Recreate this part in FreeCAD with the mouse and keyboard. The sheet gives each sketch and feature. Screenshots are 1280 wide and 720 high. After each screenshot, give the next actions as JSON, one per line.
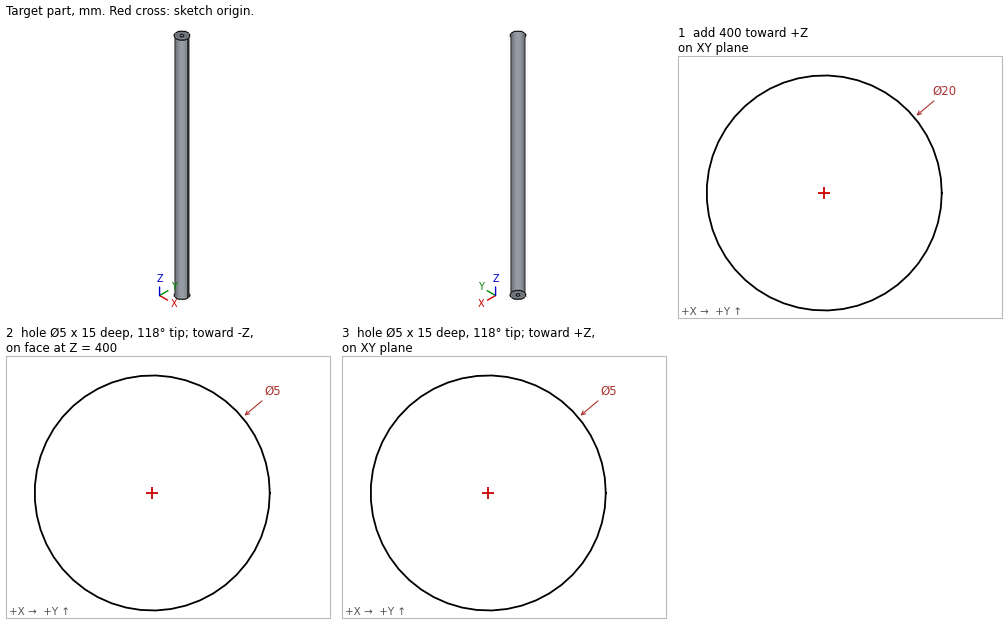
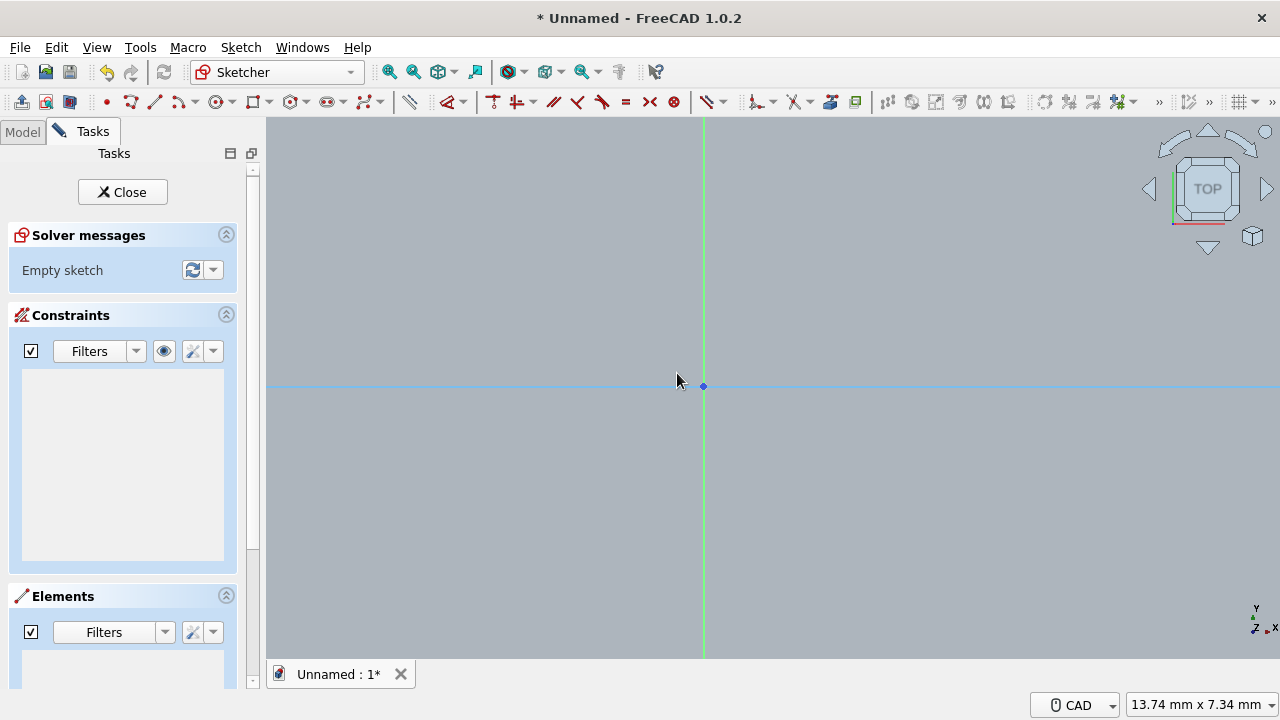
{"action": "key", "text": "g c"}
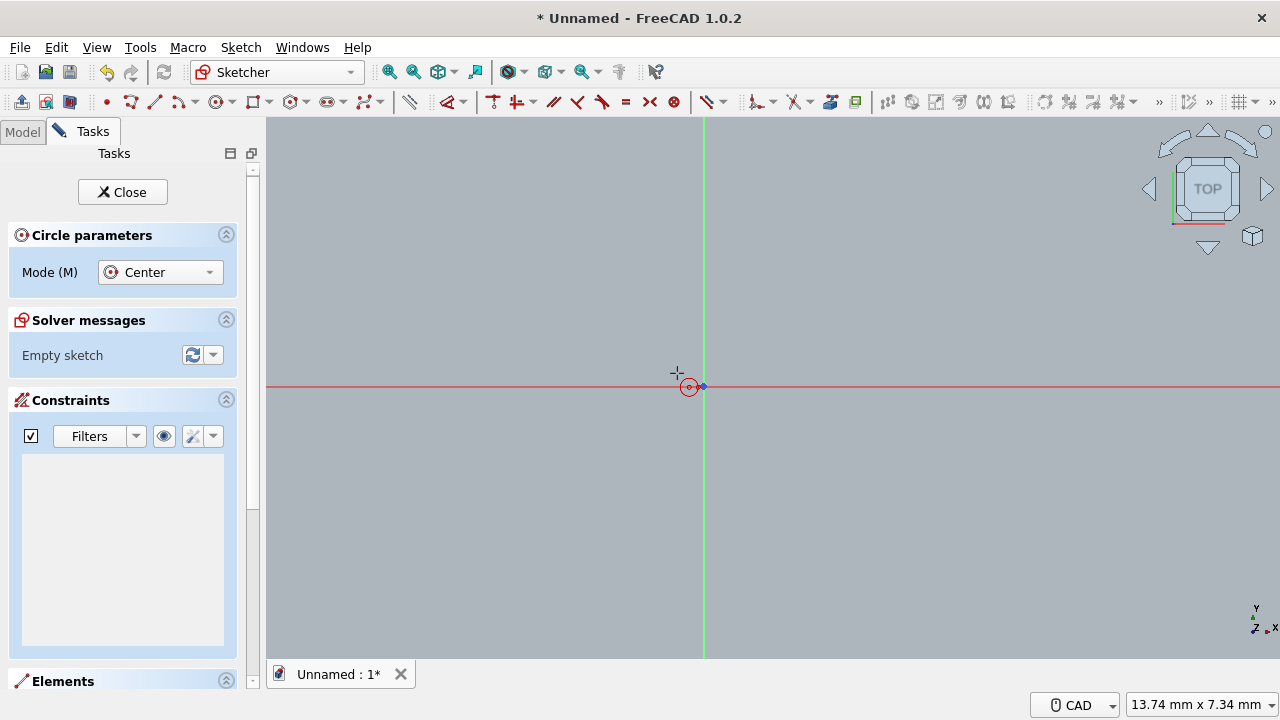
{"action": "left_click", "coordinate": [704, 387]}
{"action": "mouse_move", "coordinate": [834, 257]}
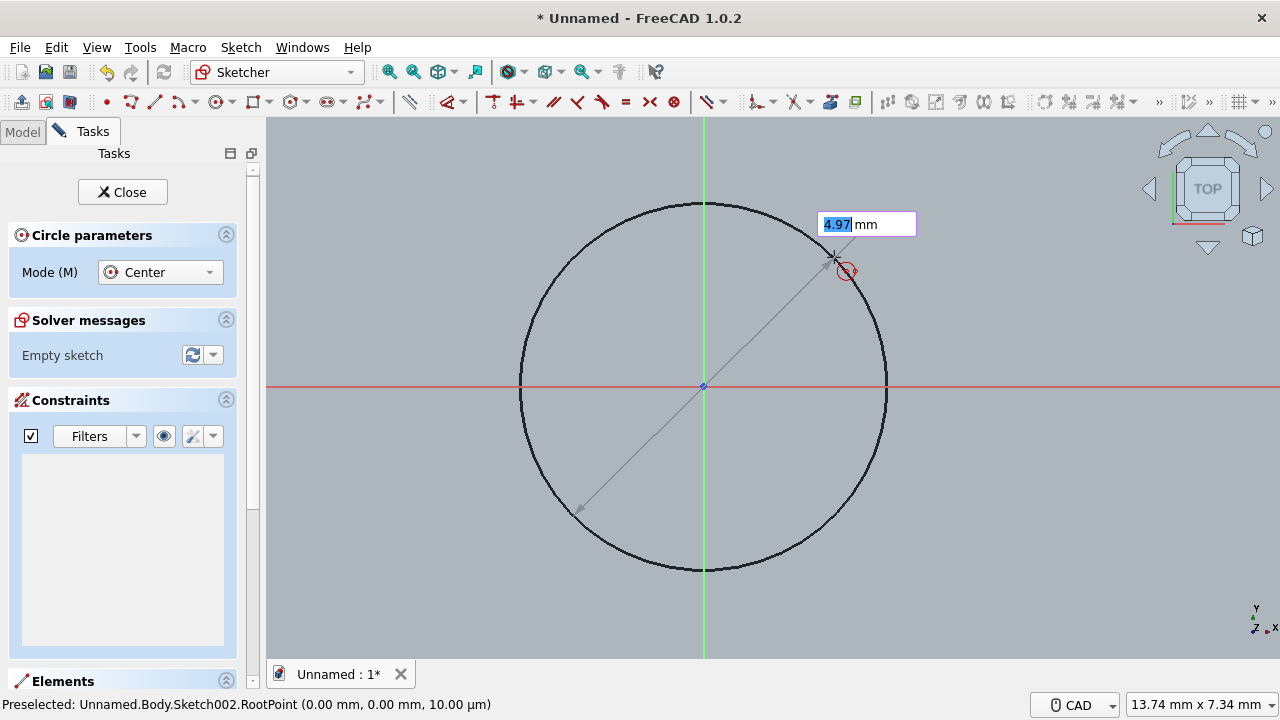
{"action": "type", "text": "5"}
{"action": "key", "text": "Return"}
{"action": "key", "text": "Escape"}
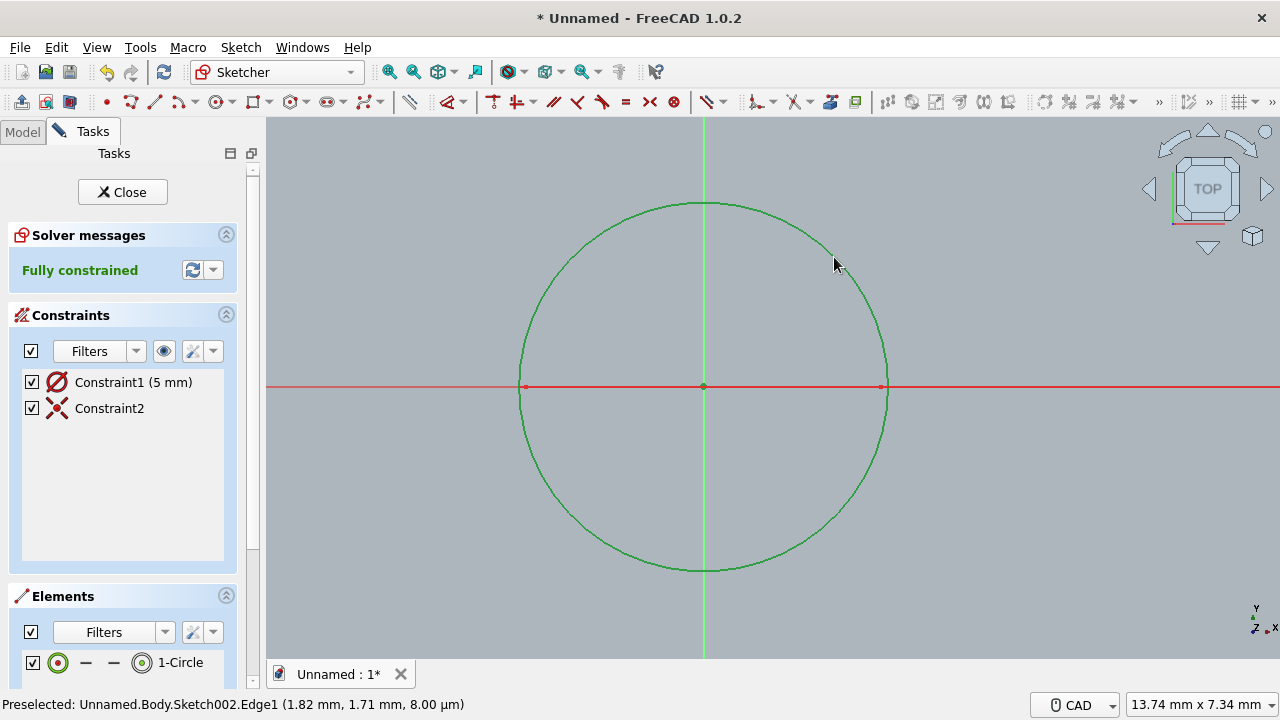
{"action": "left_click", "coordinate": [123, 192]}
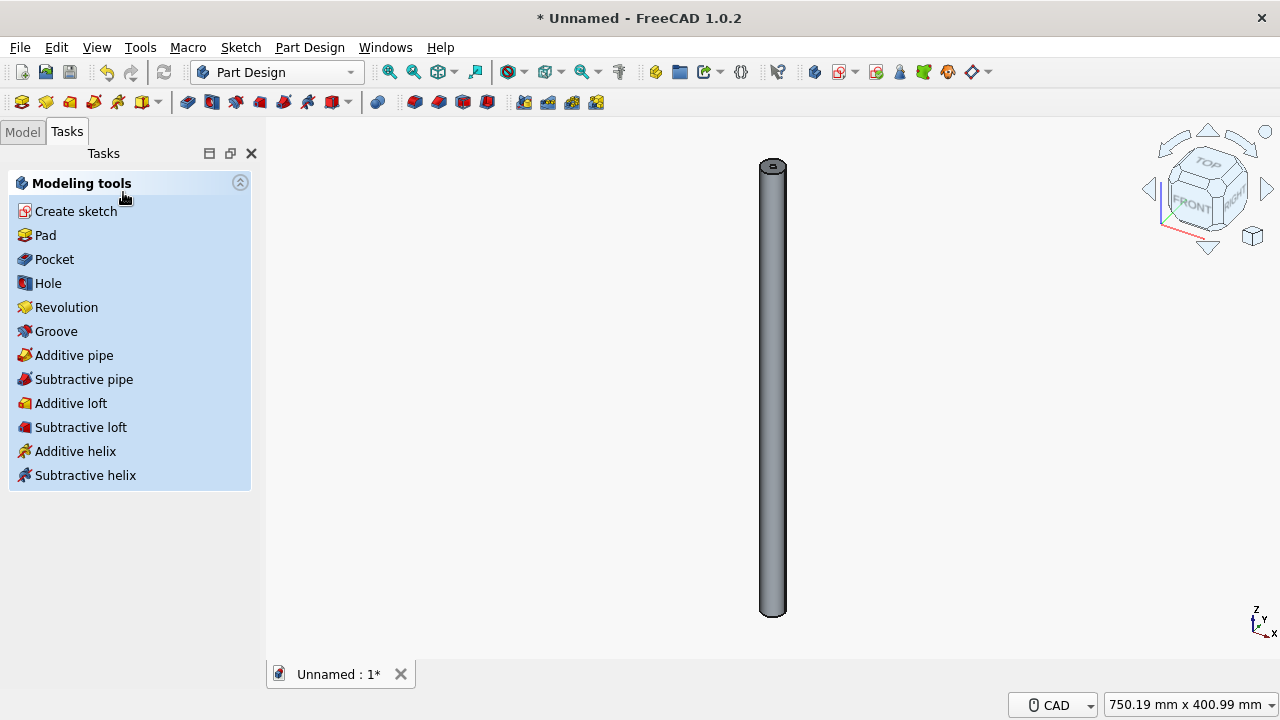
{"action": "left_click", "coordinate": [212, 102]}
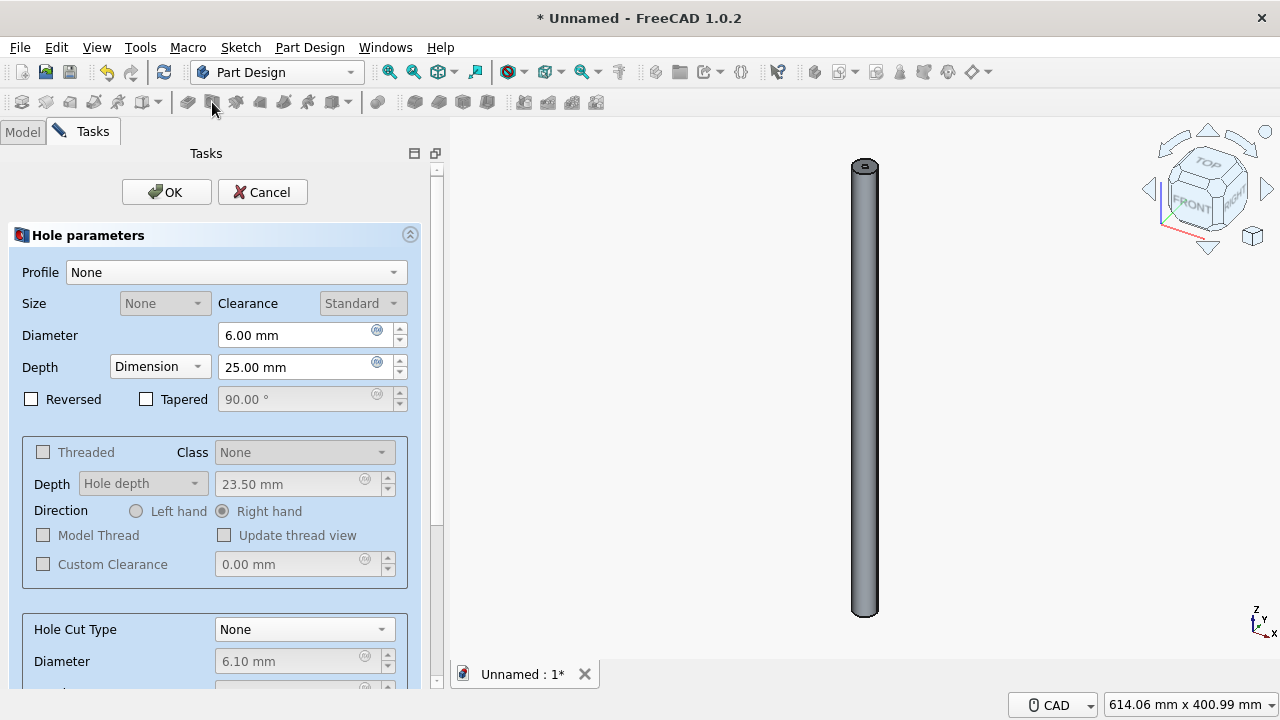
{"action": "triple_click", "coordinate": [305, 335]}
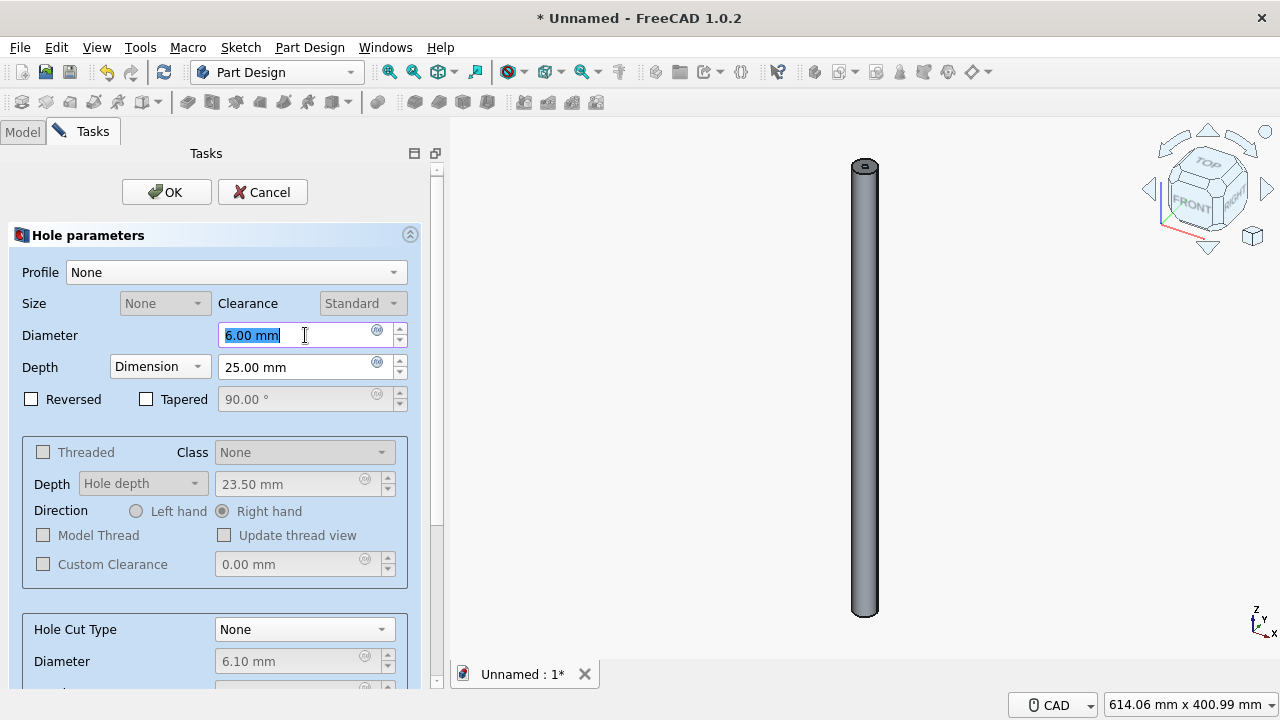
{"action": "type", "text": "5"}
{"action": "key", "text": "Tab"}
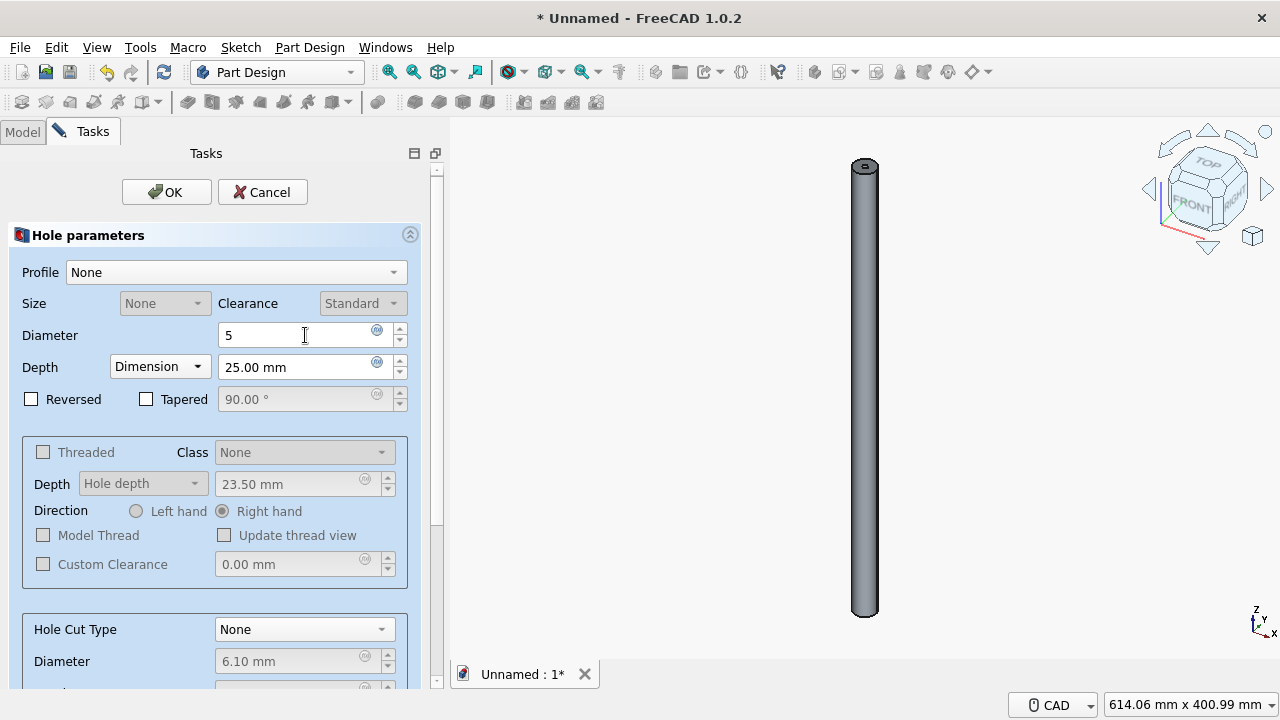
{"action": "triple_click", "coordinate": [305, 367]}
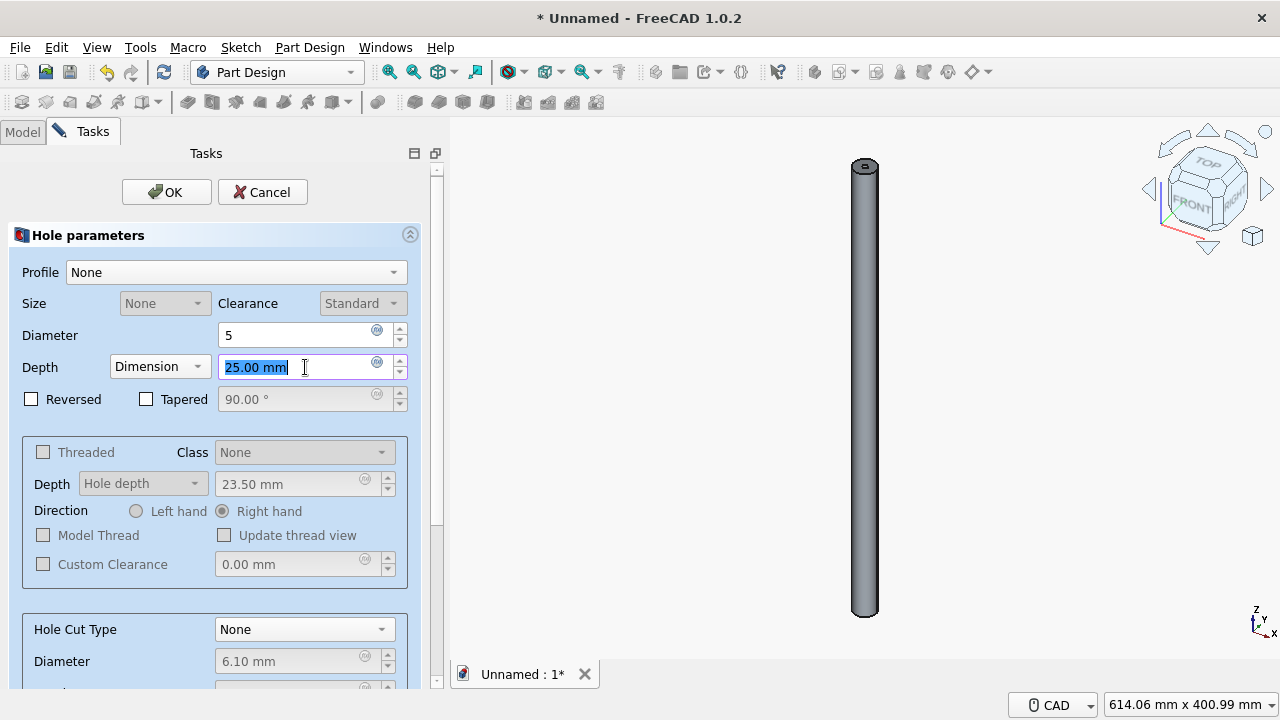
{"action": "type", "text": "15"}
{"action": "key", "text": "Tab"}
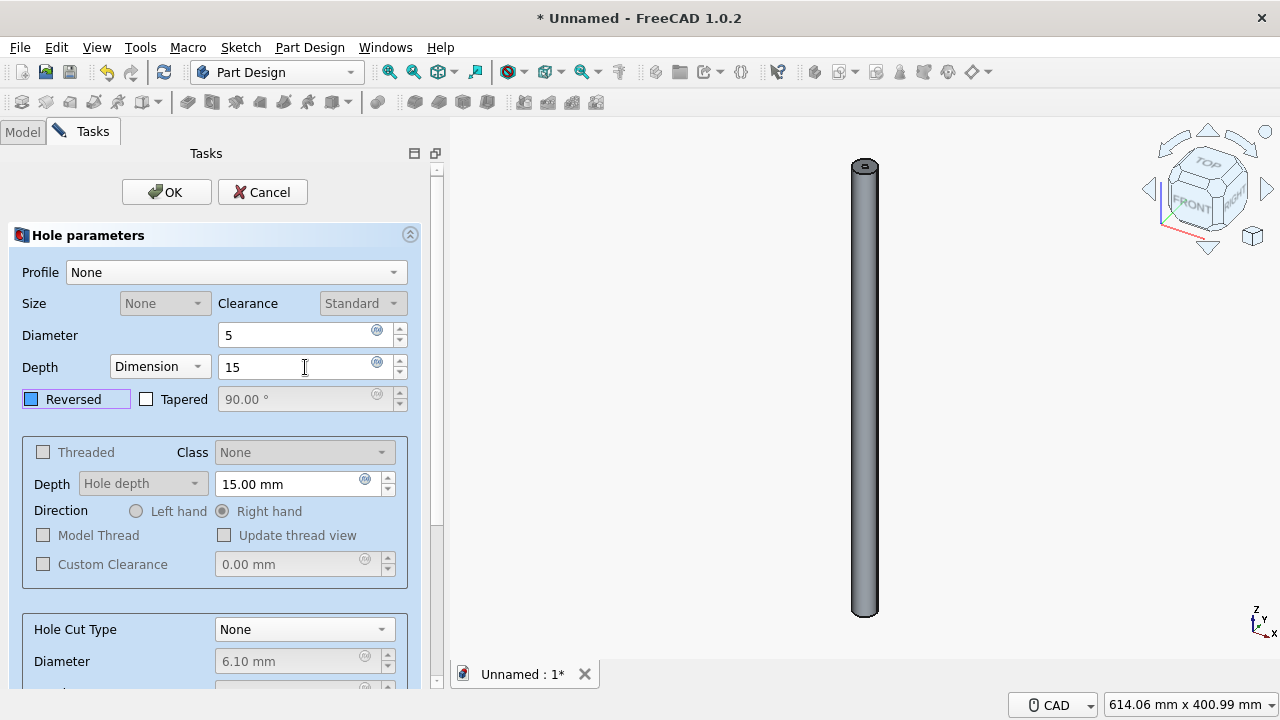
{"action": "left_click", "coordinate": [30, 399]}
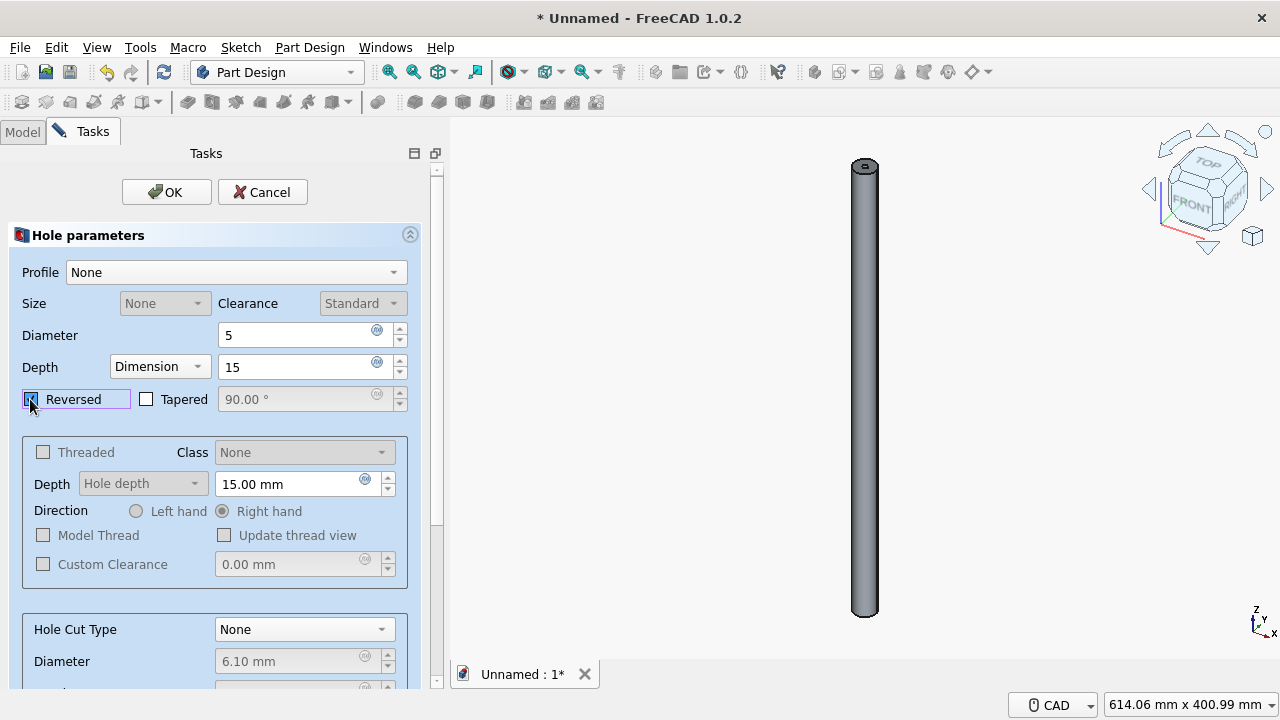
{"action": "left_click", "coordinate": [167, 192]}